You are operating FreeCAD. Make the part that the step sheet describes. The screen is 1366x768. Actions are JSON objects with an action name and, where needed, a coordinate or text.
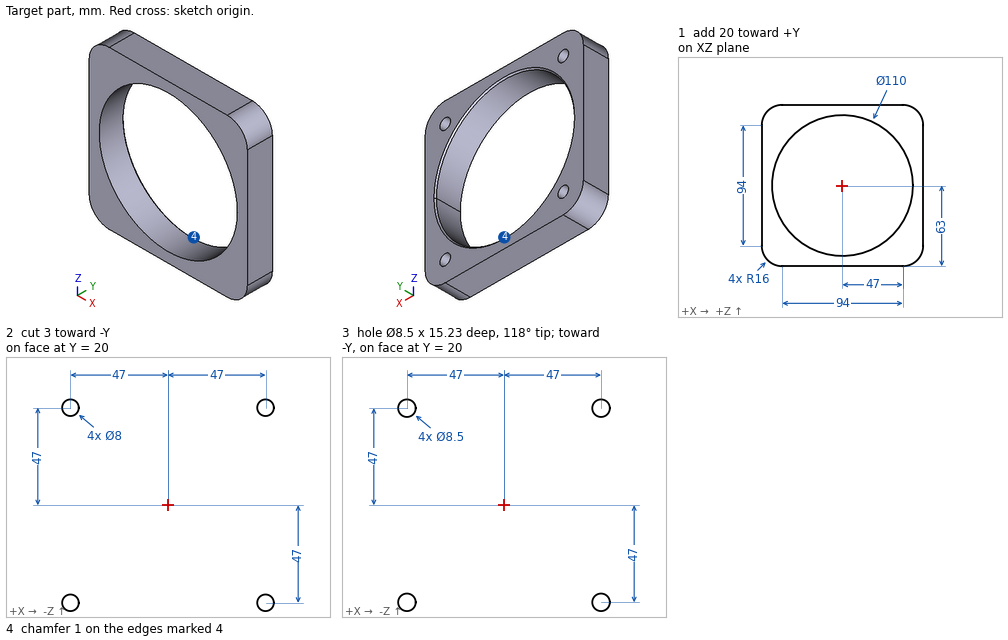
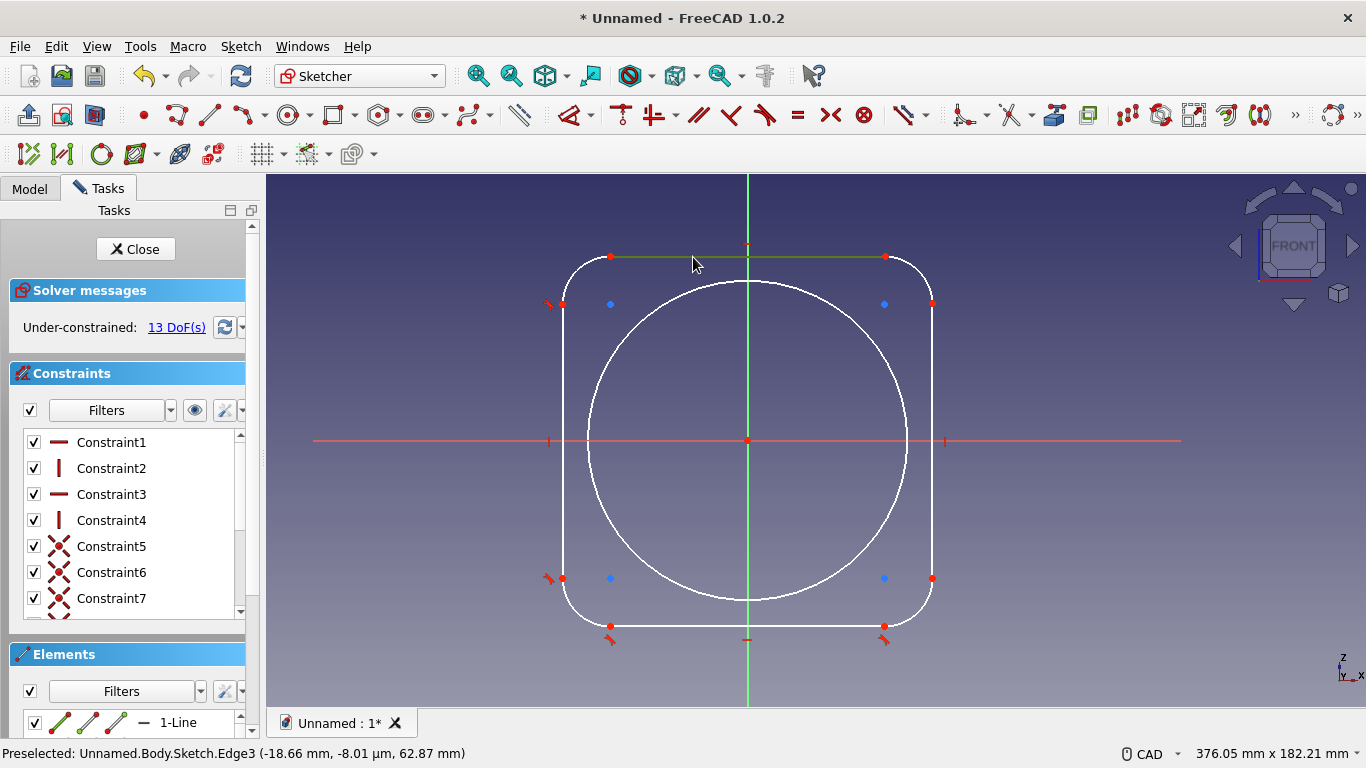
{"action": "left_click", "coordinate": [589, 262]}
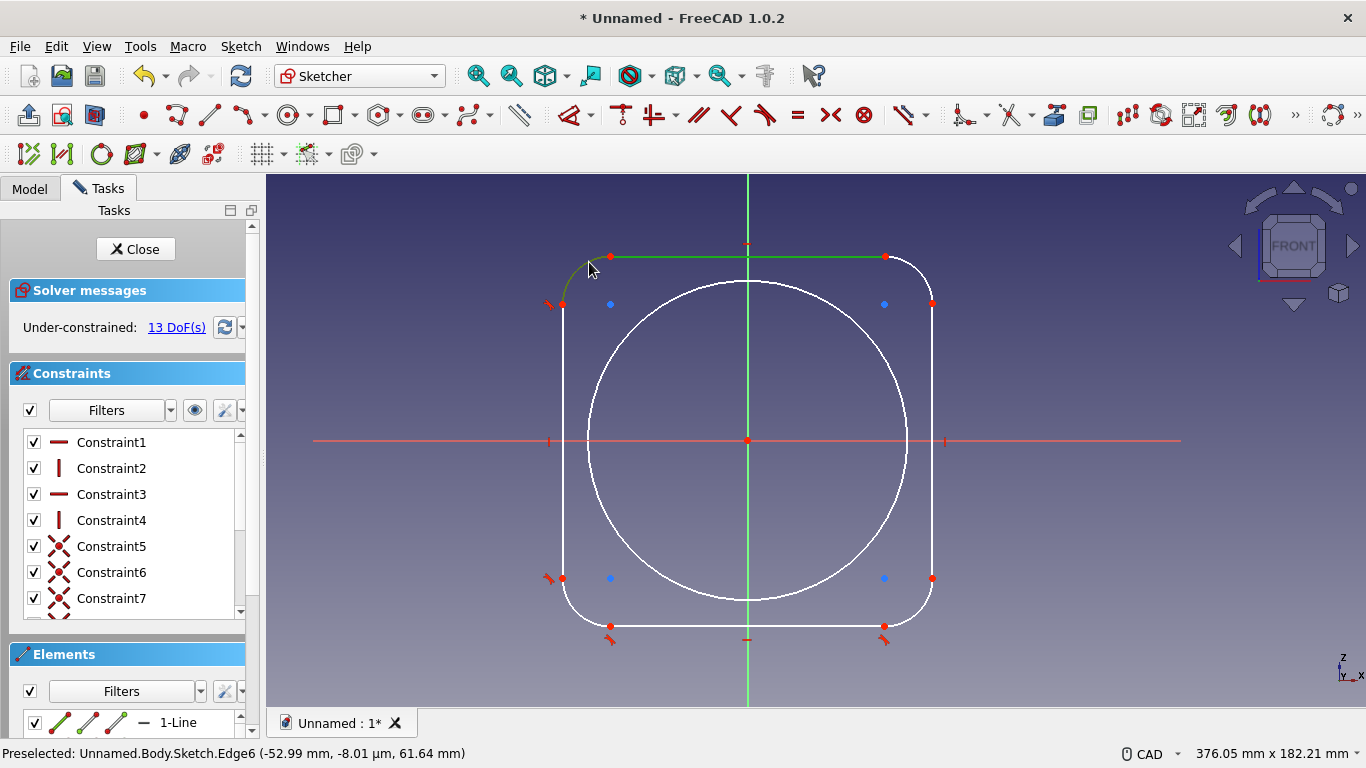
{"action": "left_click", "coordinate": [765, 116]}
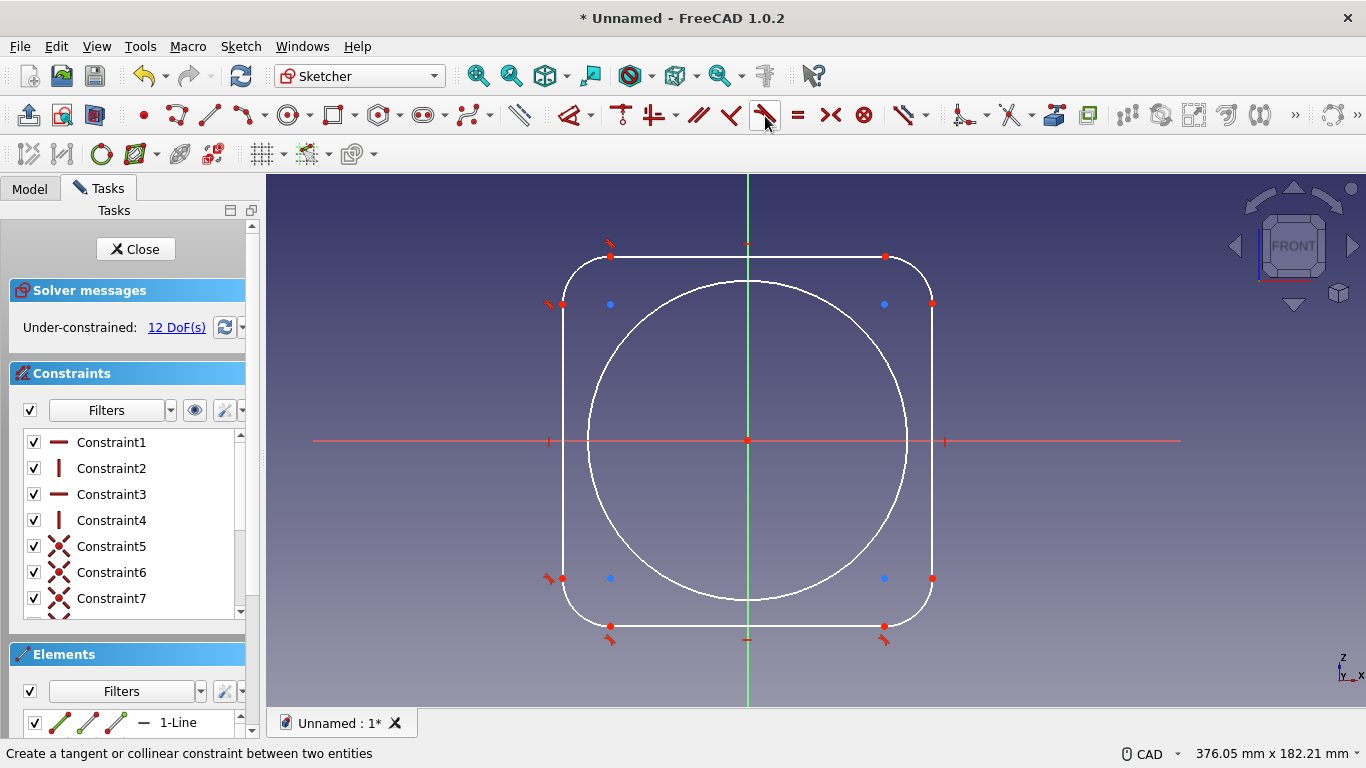
{"action": "left_click", "coordinate": [693, 257]}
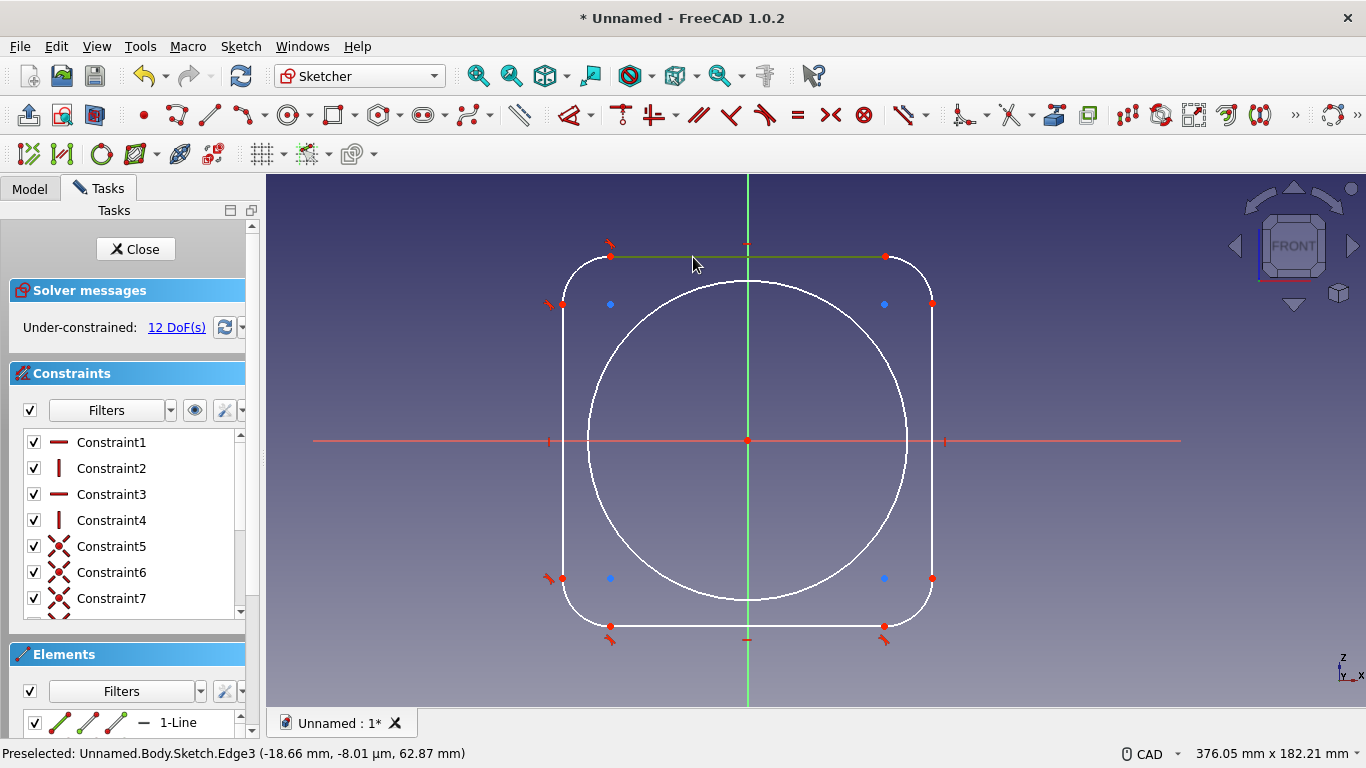
{"action": "left_click", "coordinate": [927, 283]}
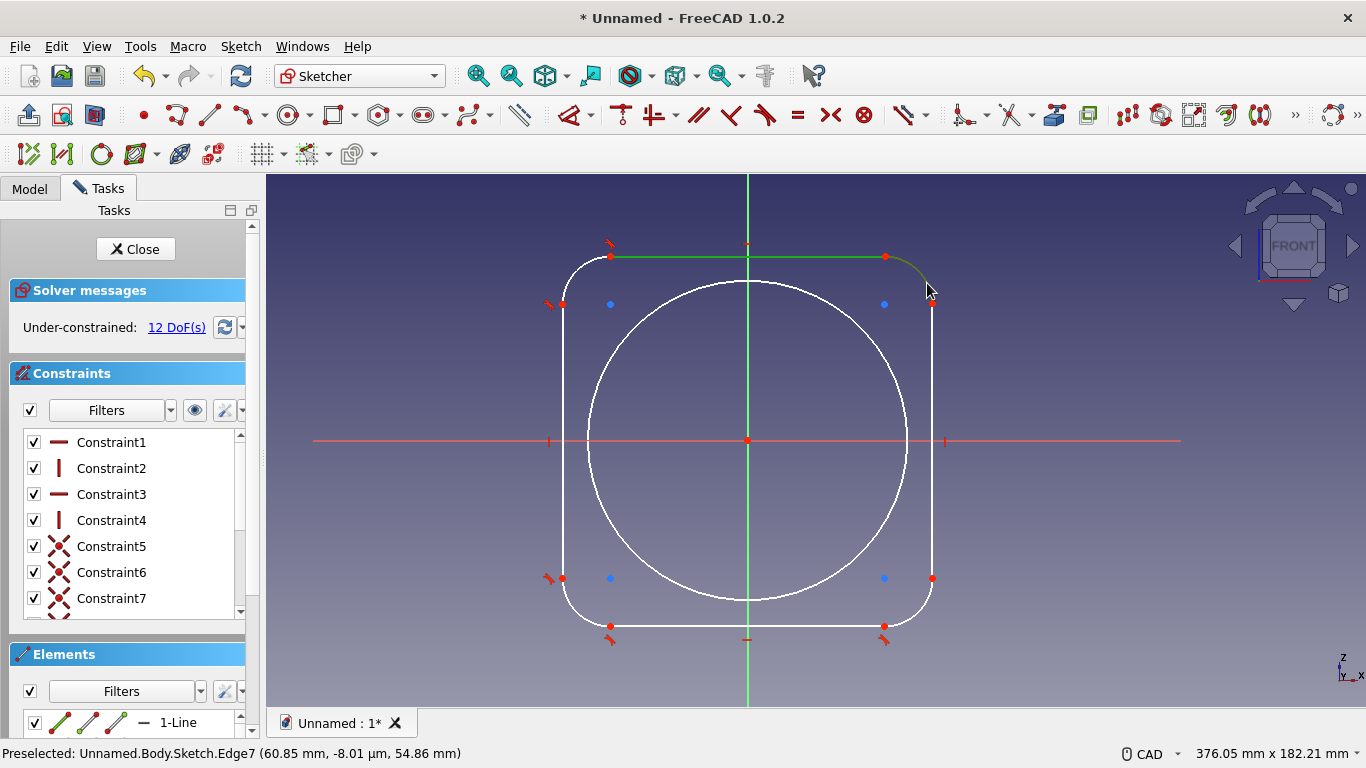
{"action": "key", "text": "t"}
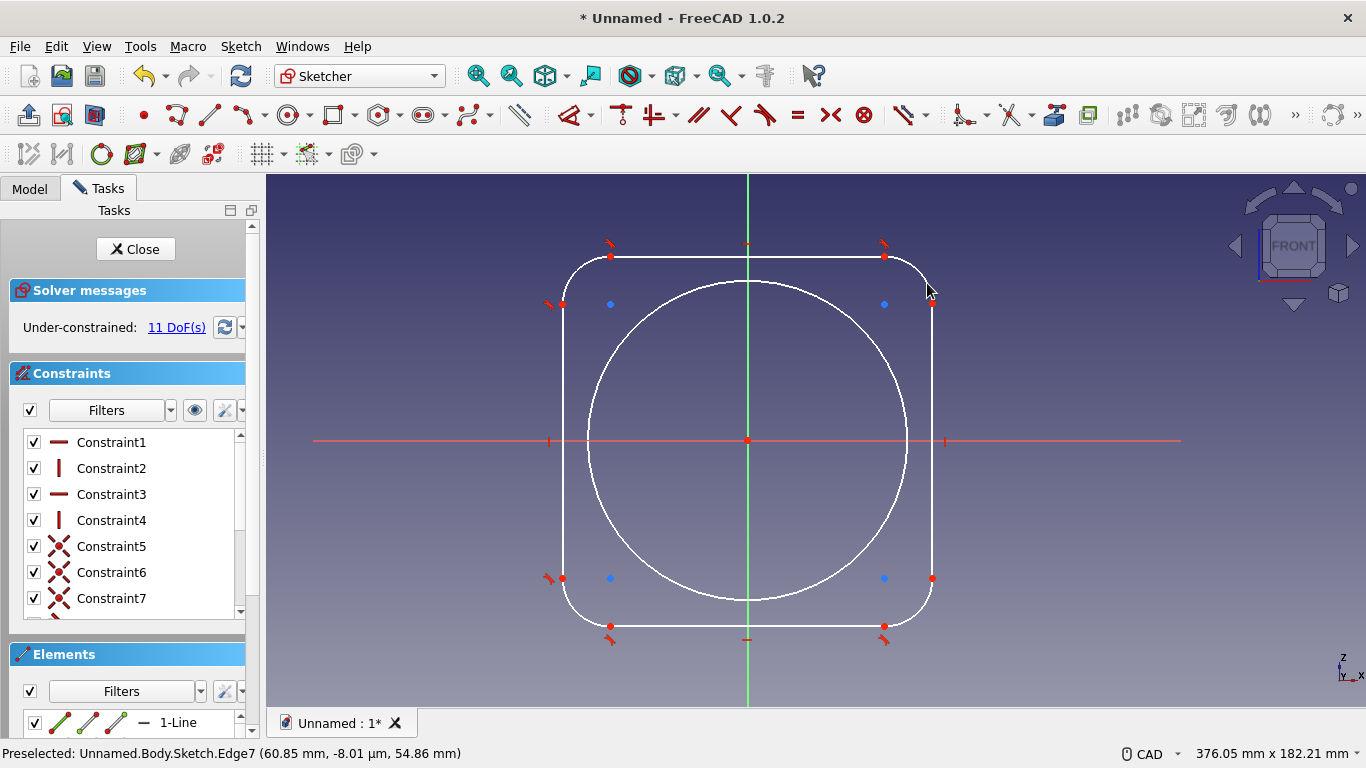
{"action": "left_click", "coordinate": [932, 386]}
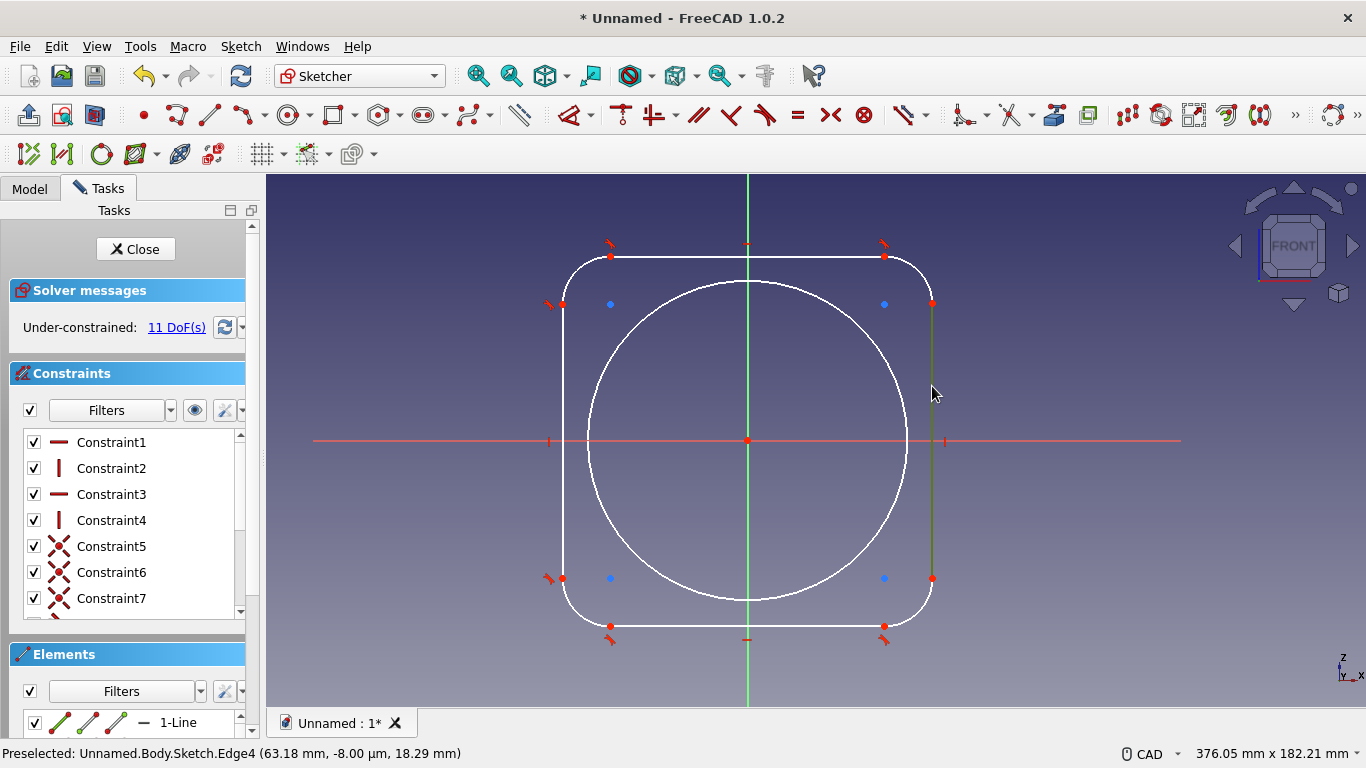
{"action": "left_click", "coordinate": [927, 282]}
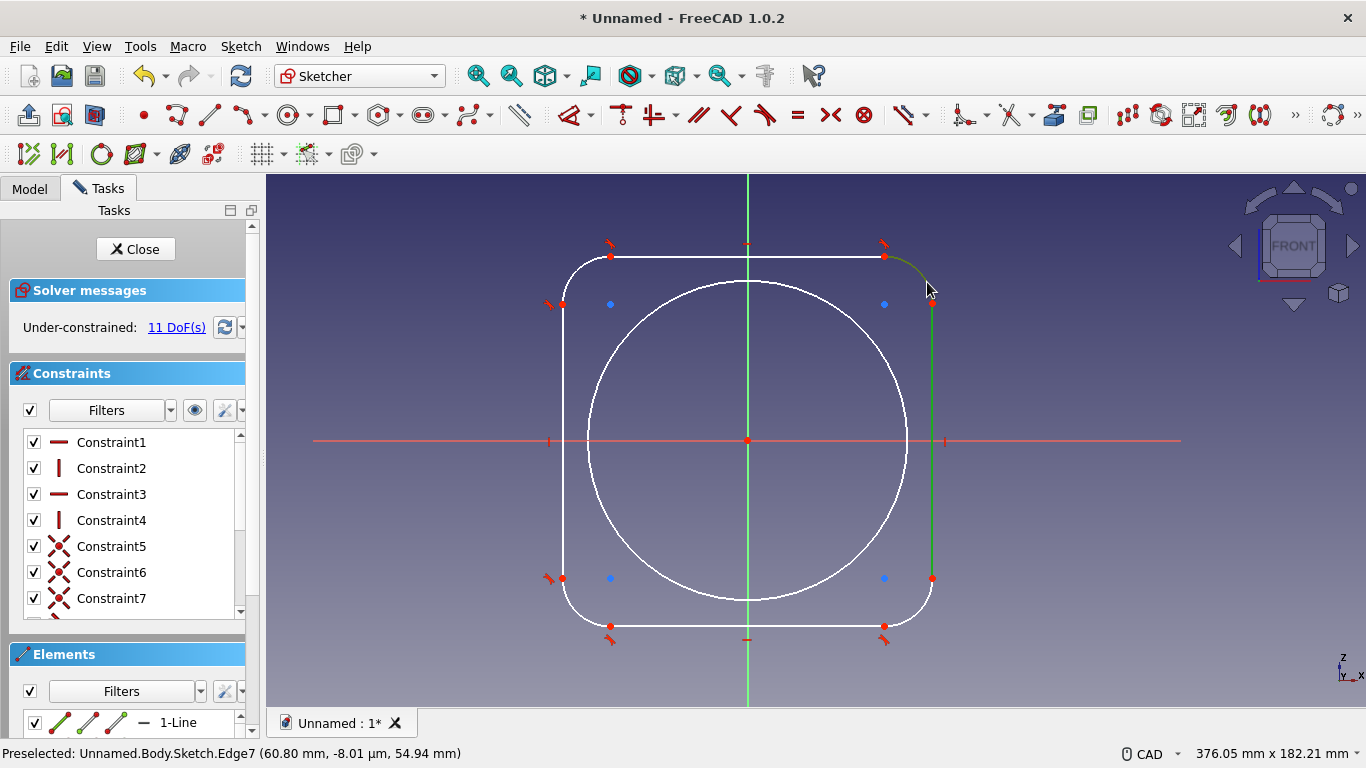
{"action": "key", "text": "t"}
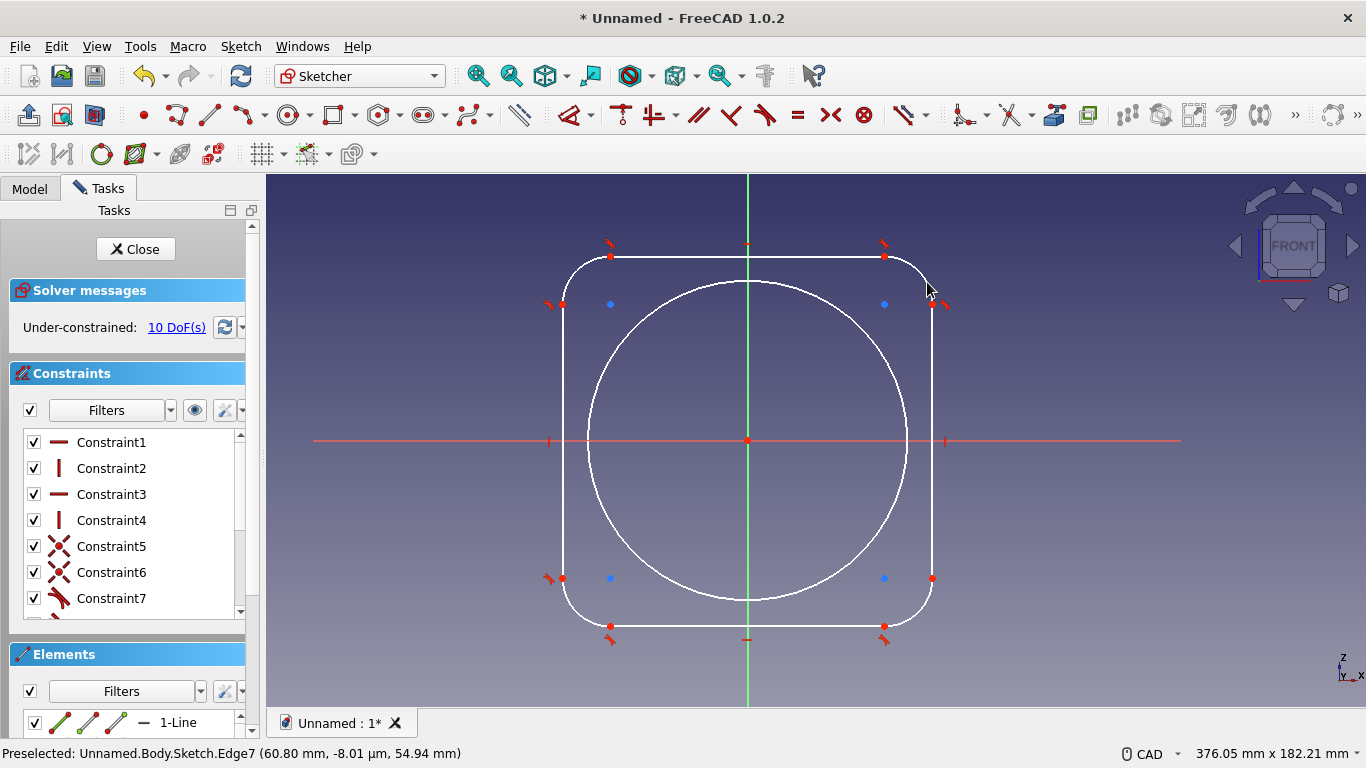
{"action": "left_click", "coordinate": [932, 387]}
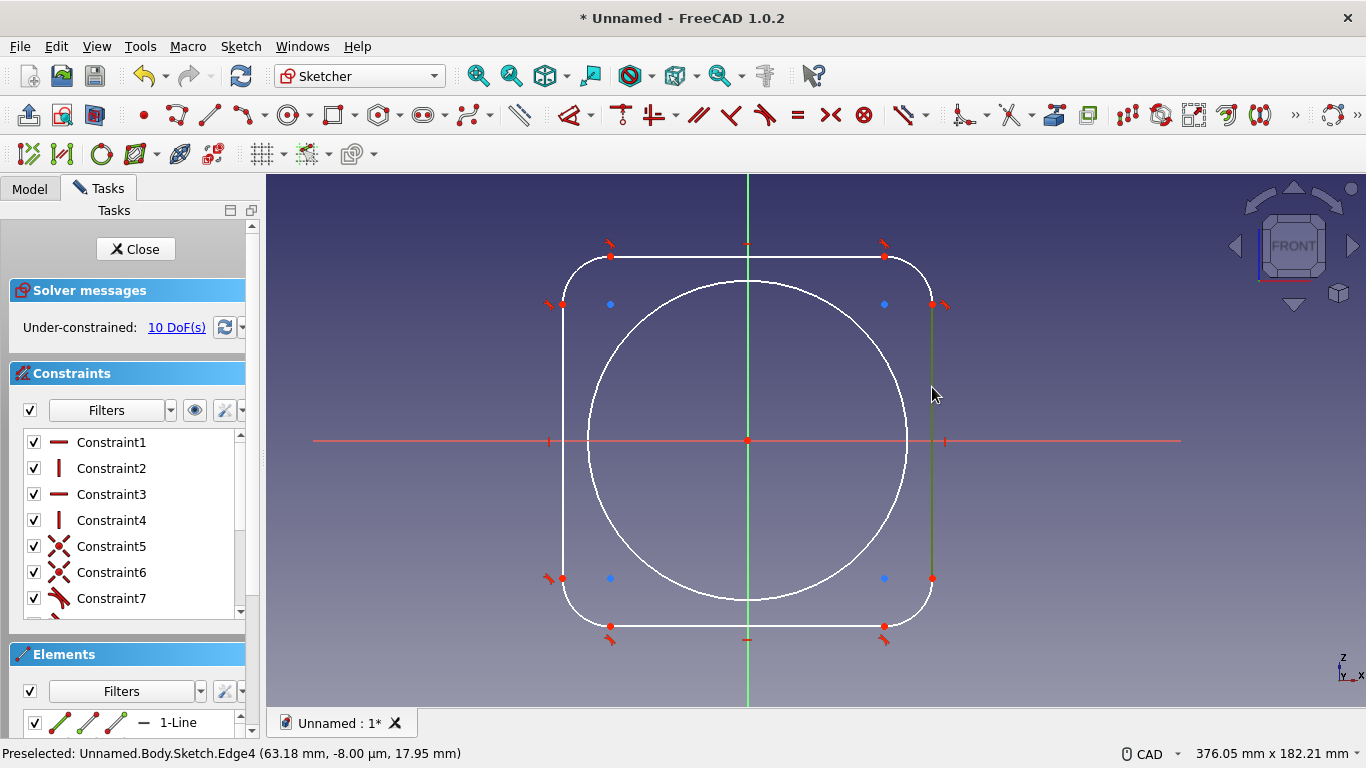
{"action": "left_click", "coordinate": [906, 621]}